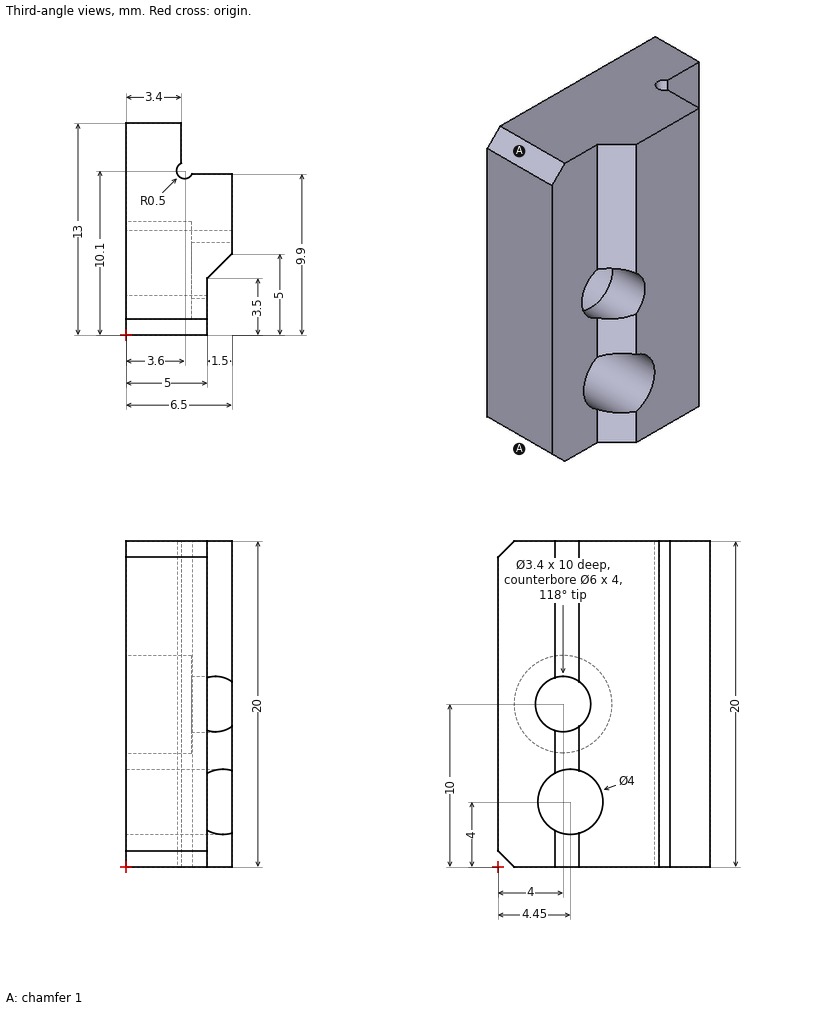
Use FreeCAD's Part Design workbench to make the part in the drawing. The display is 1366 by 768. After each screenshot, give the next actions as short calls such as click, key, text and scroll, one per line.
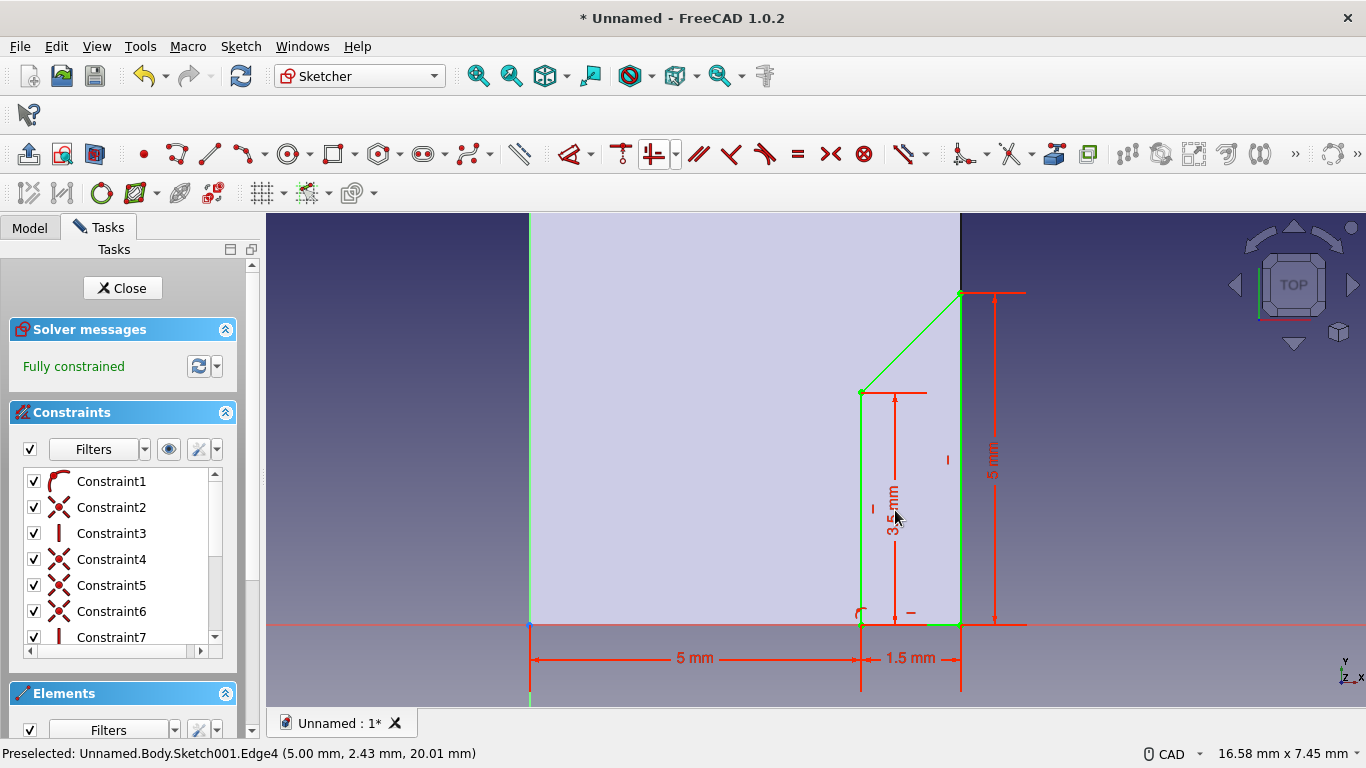
click(123, 288)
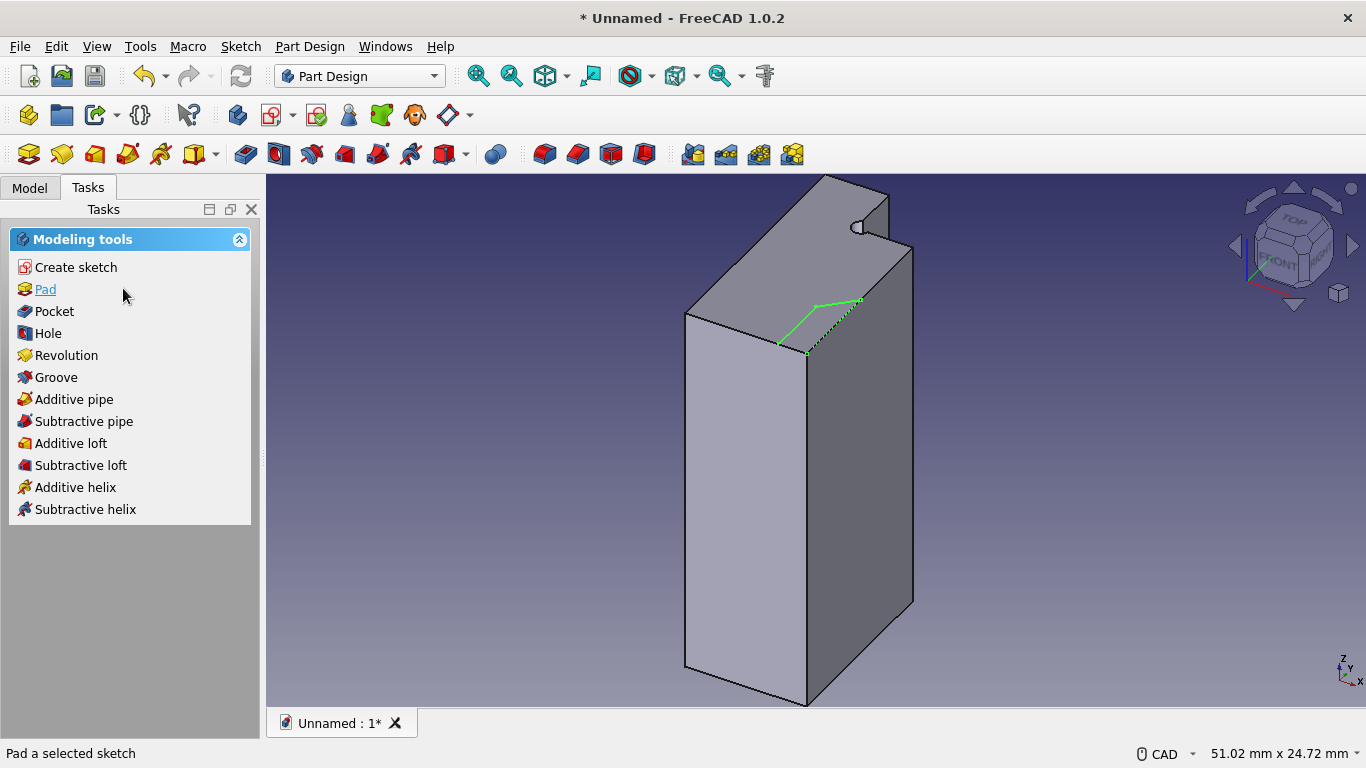
click(246, 154)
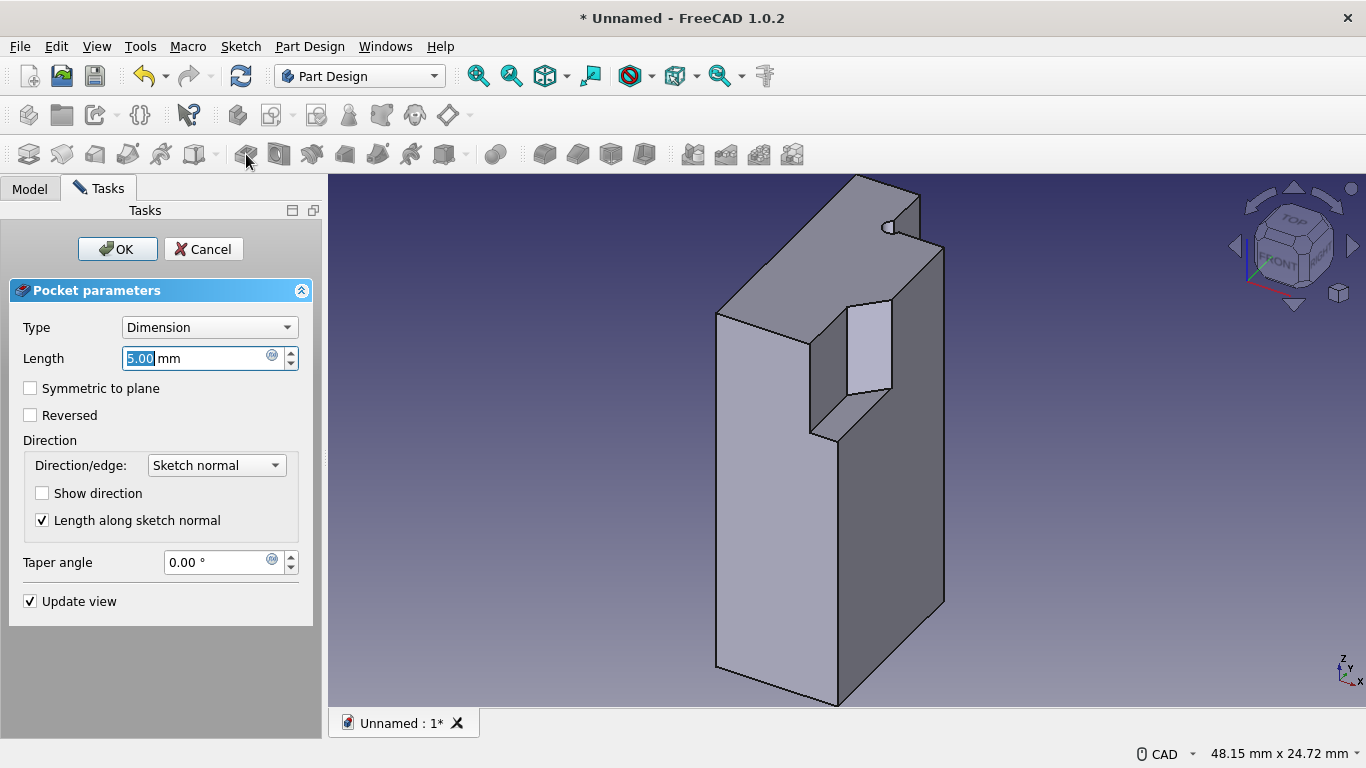
text(20)
key(Tab)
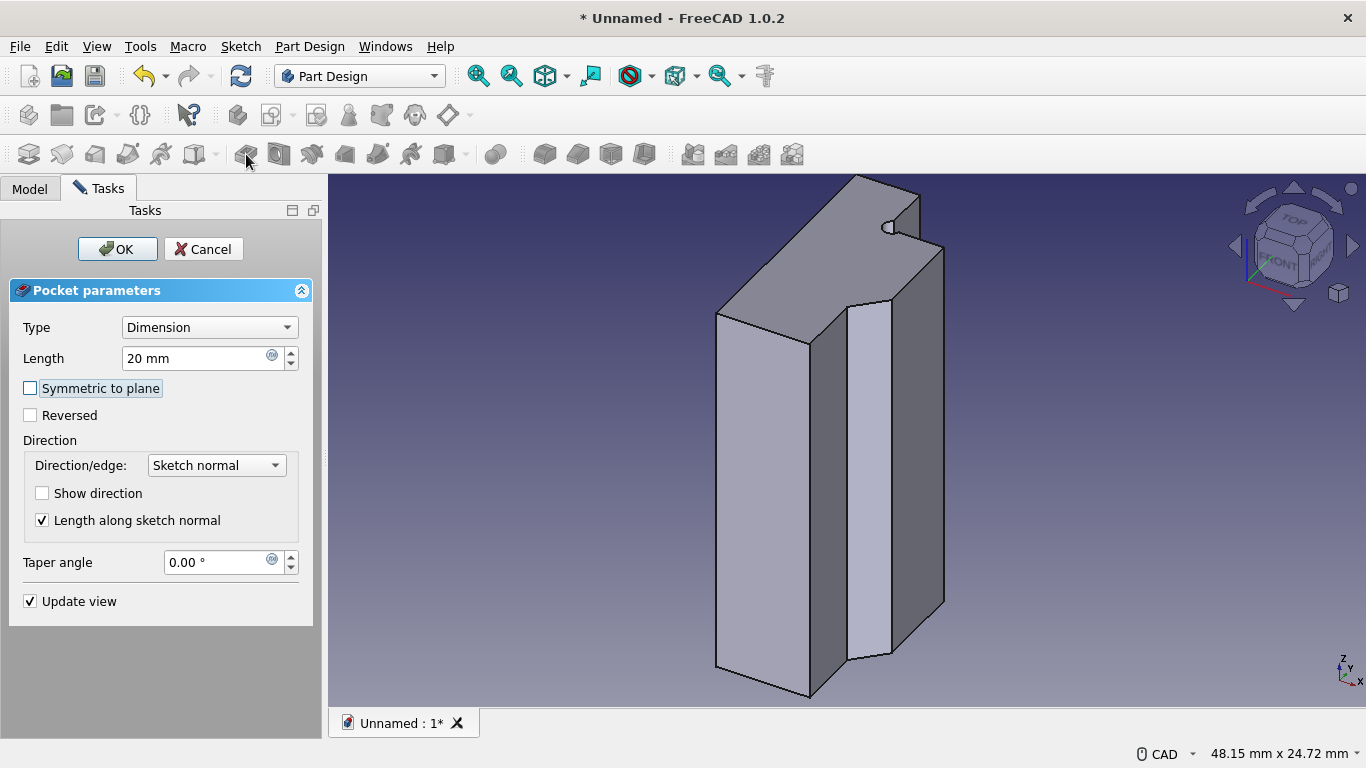
click(118, 249)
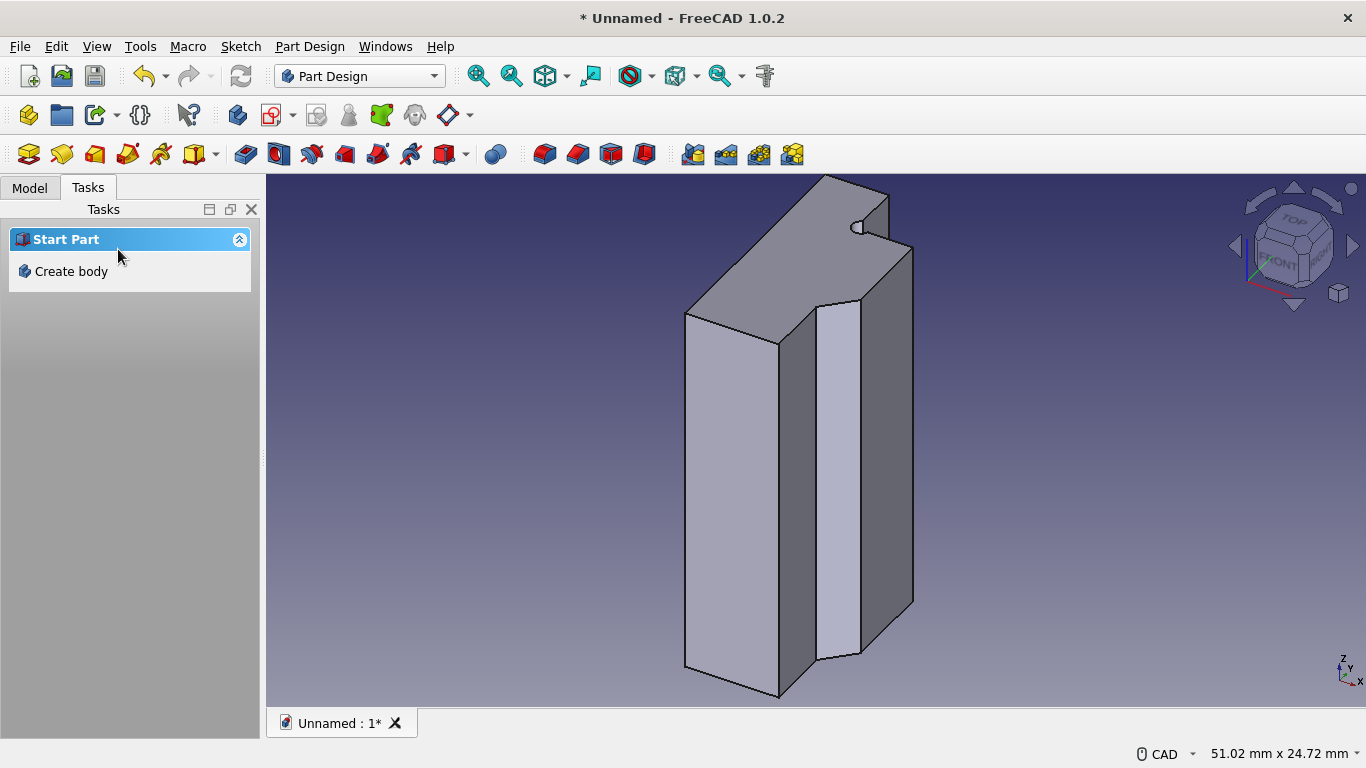
click(479, 76)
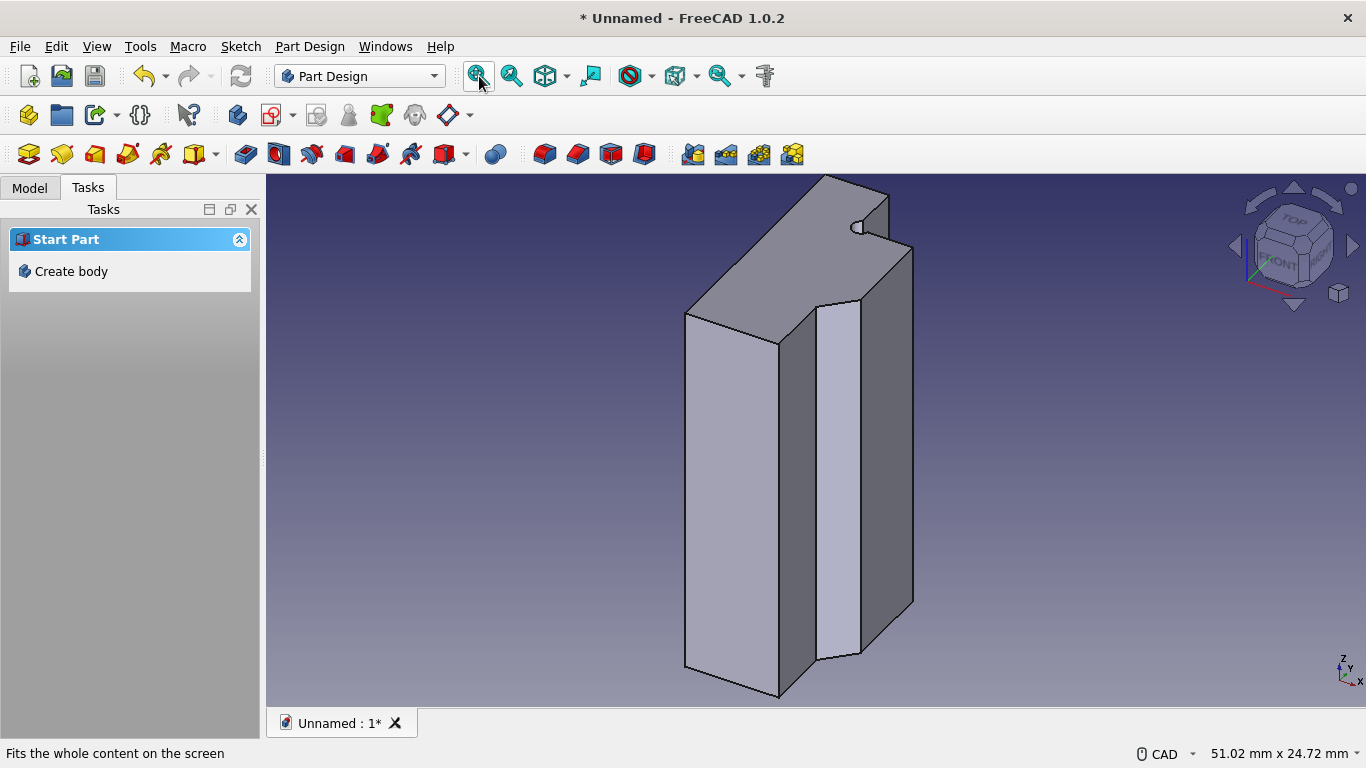
click(270, 116)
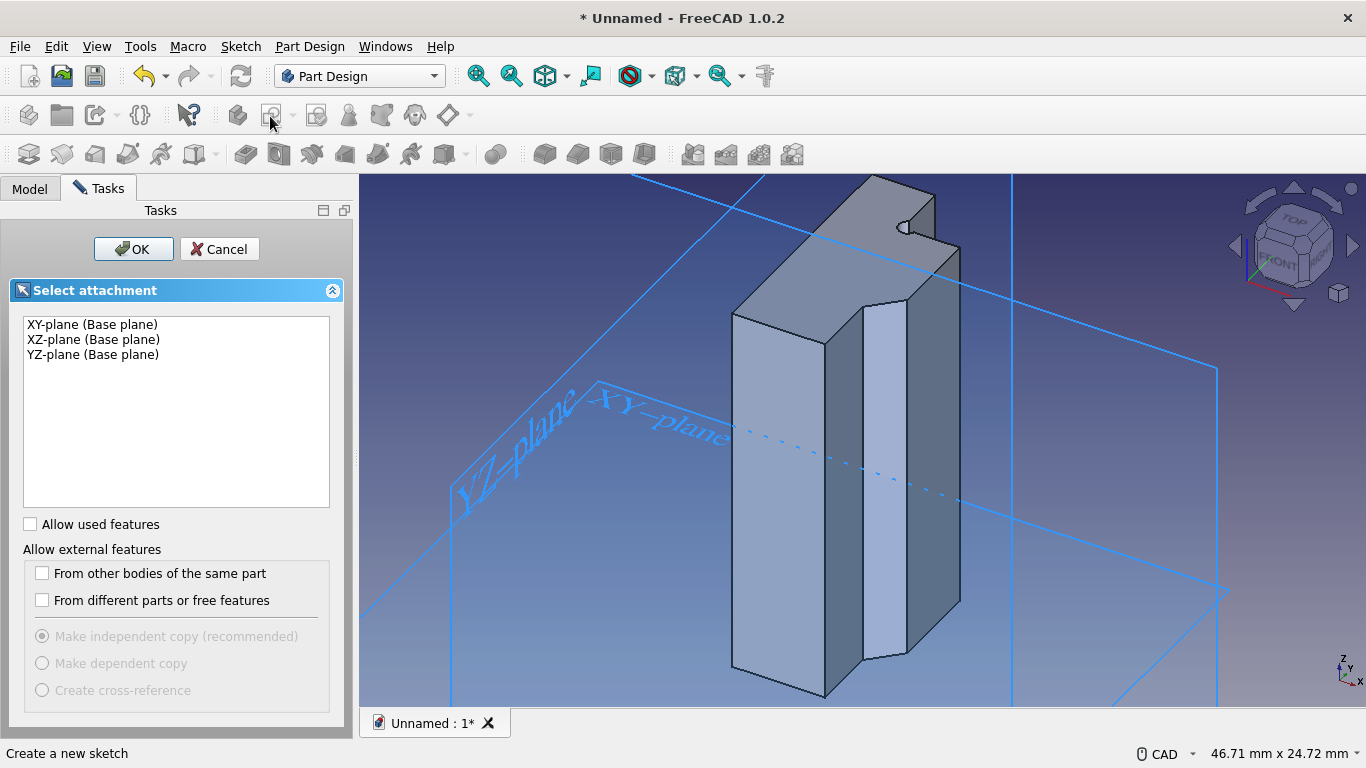
click(84, 354)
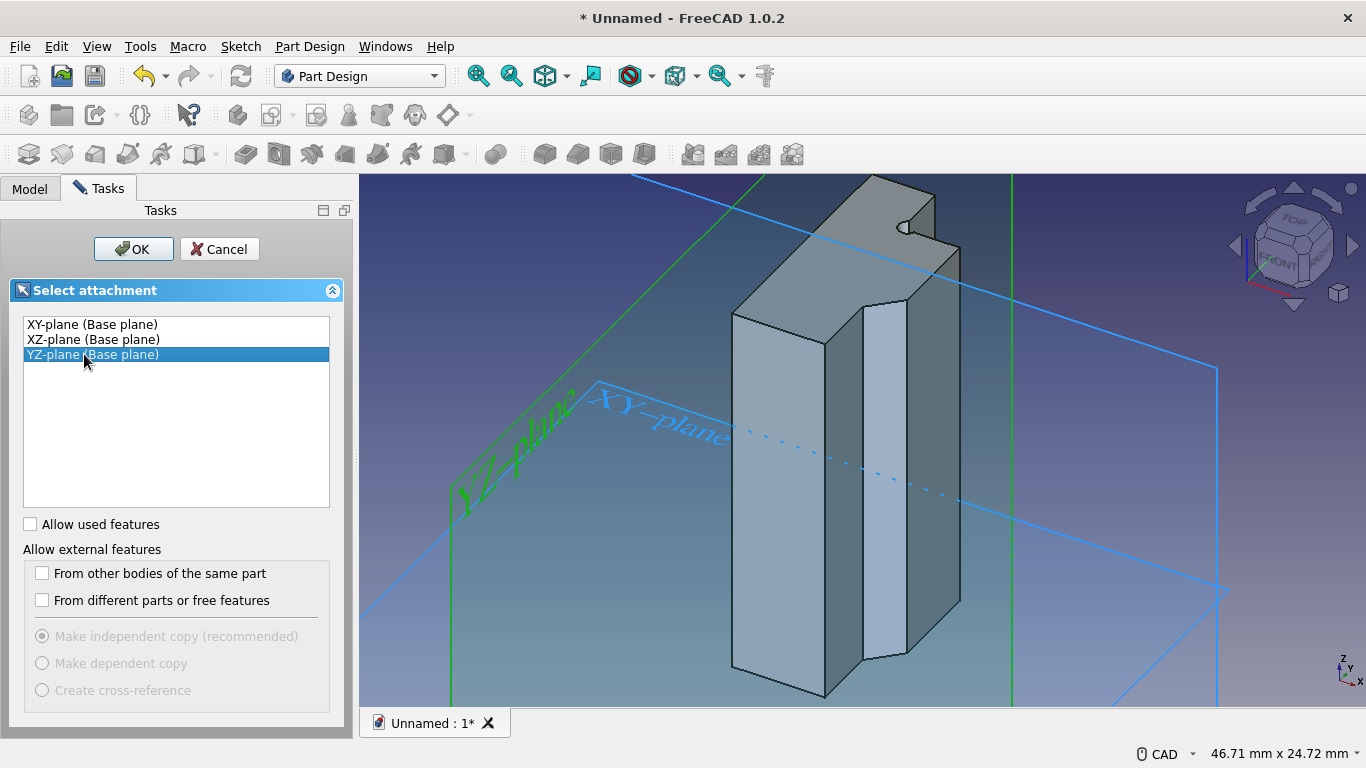
click(134, 249)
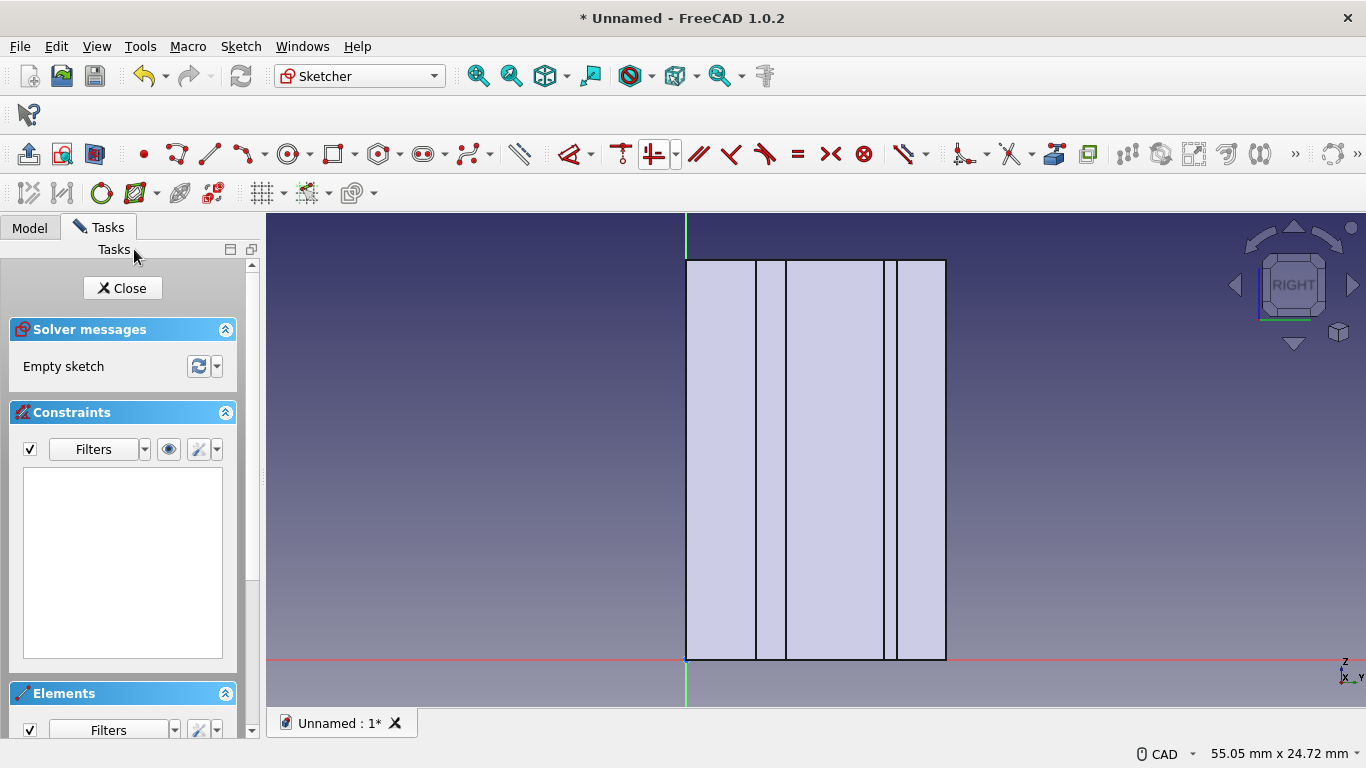
click(95, 154)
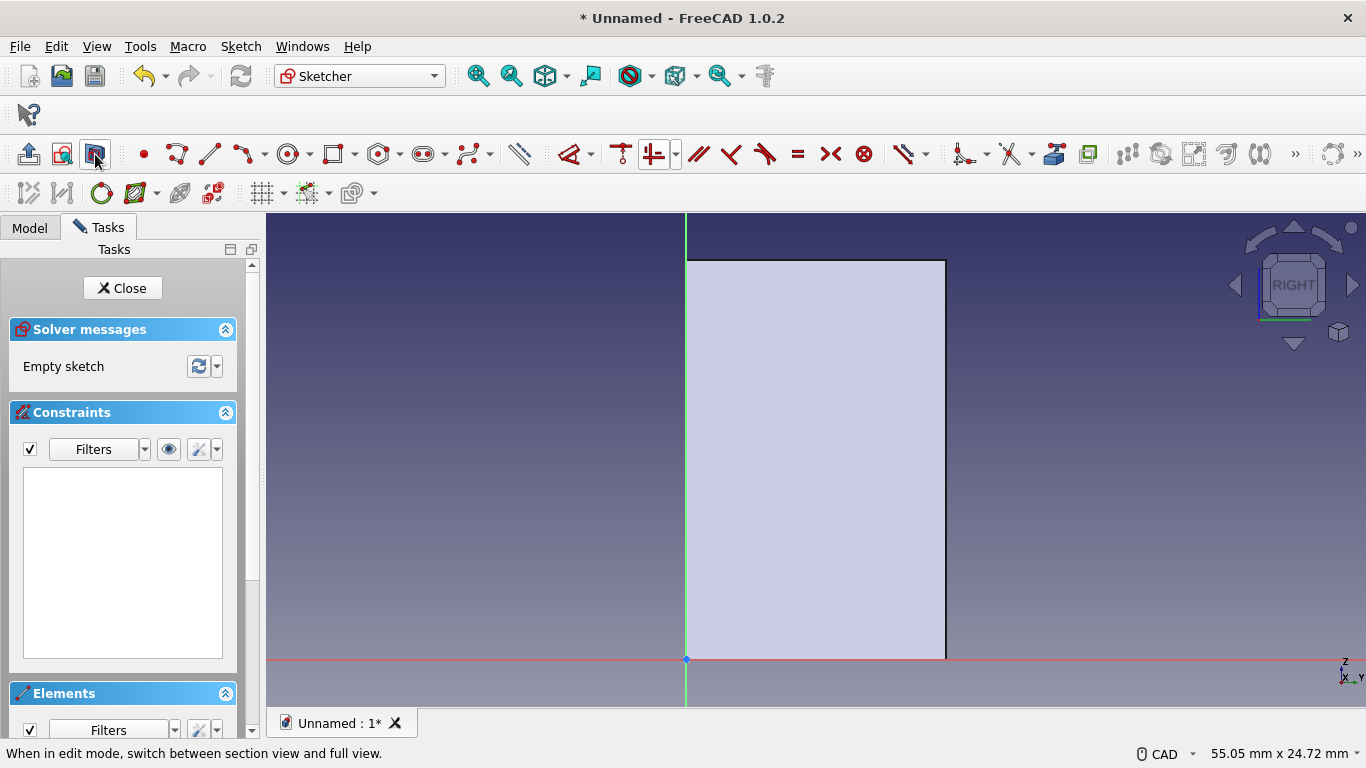
scroll(771, 460, up, 8)